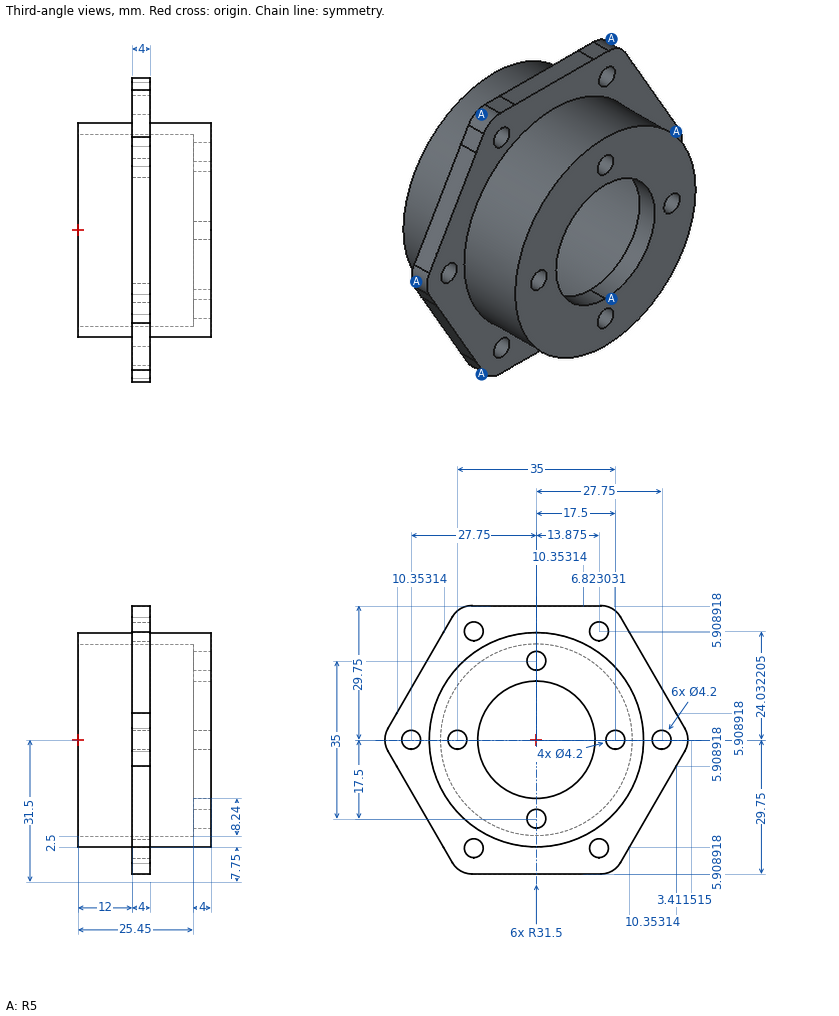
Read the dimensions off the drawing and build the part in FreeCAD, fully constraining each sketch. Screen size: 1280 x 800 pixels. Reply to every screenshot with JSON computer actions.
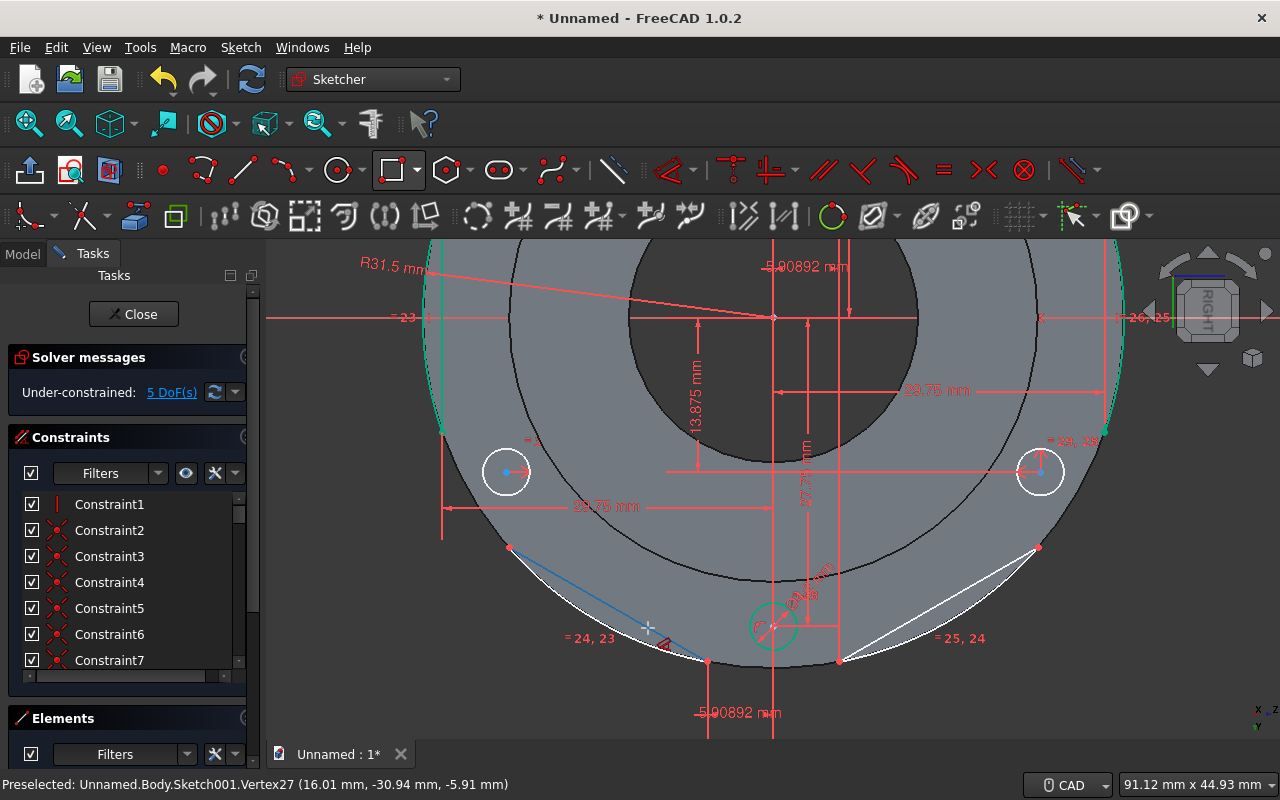
{"action": "left_click", "coordinate": [648, 628]}
{"action": "left_click", "coordinate": [475, 605]}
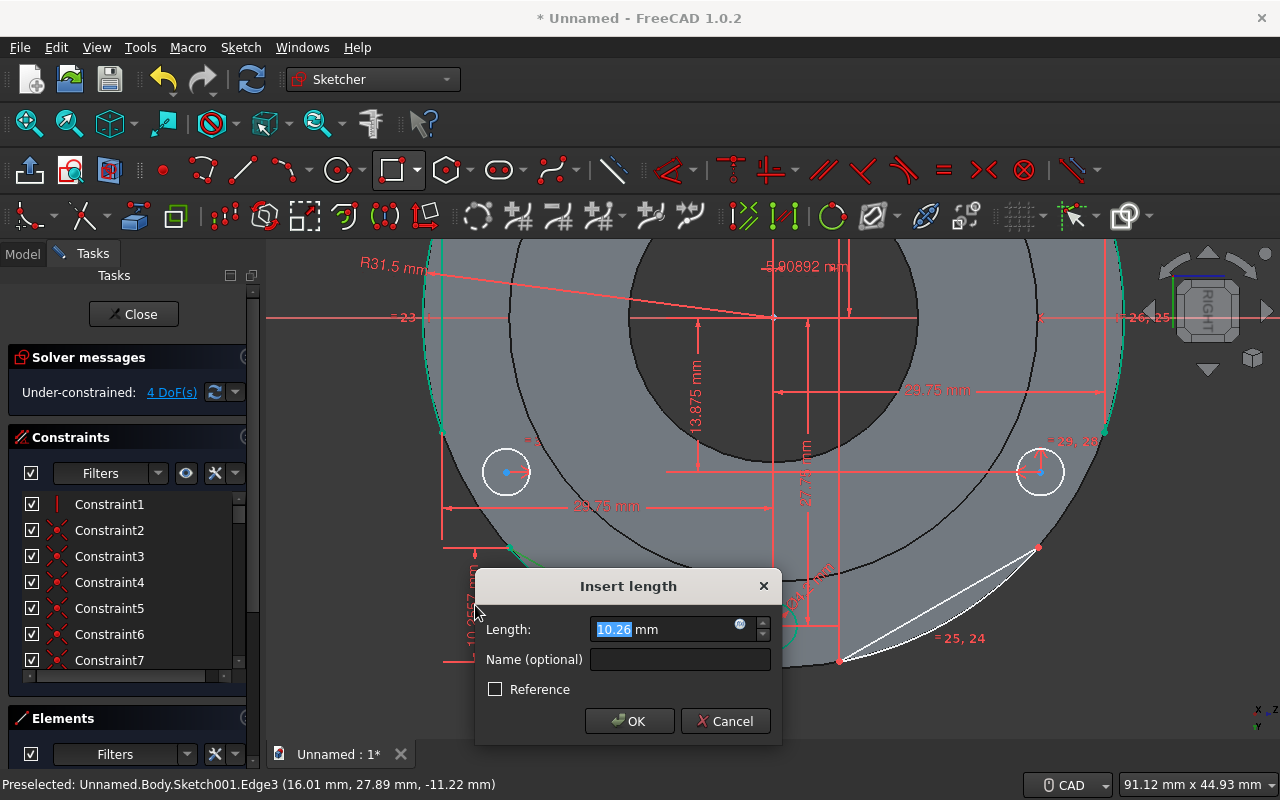
{"action": "type", "text": "10.35314"}
{"action": "key", "text": "Return"}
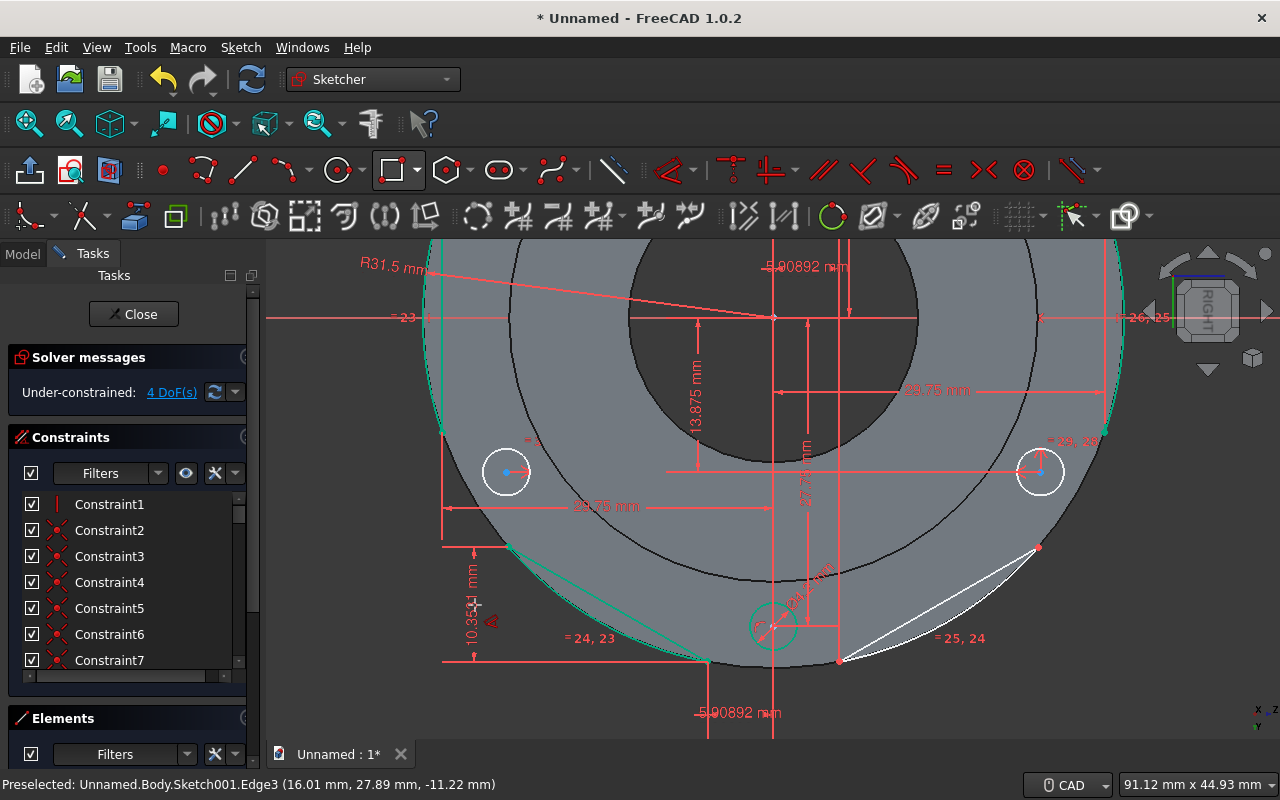
{"action": "left_click", "coordinate": [978, 582]}
{"action": "left_click", "coordinate": [1072, 605]}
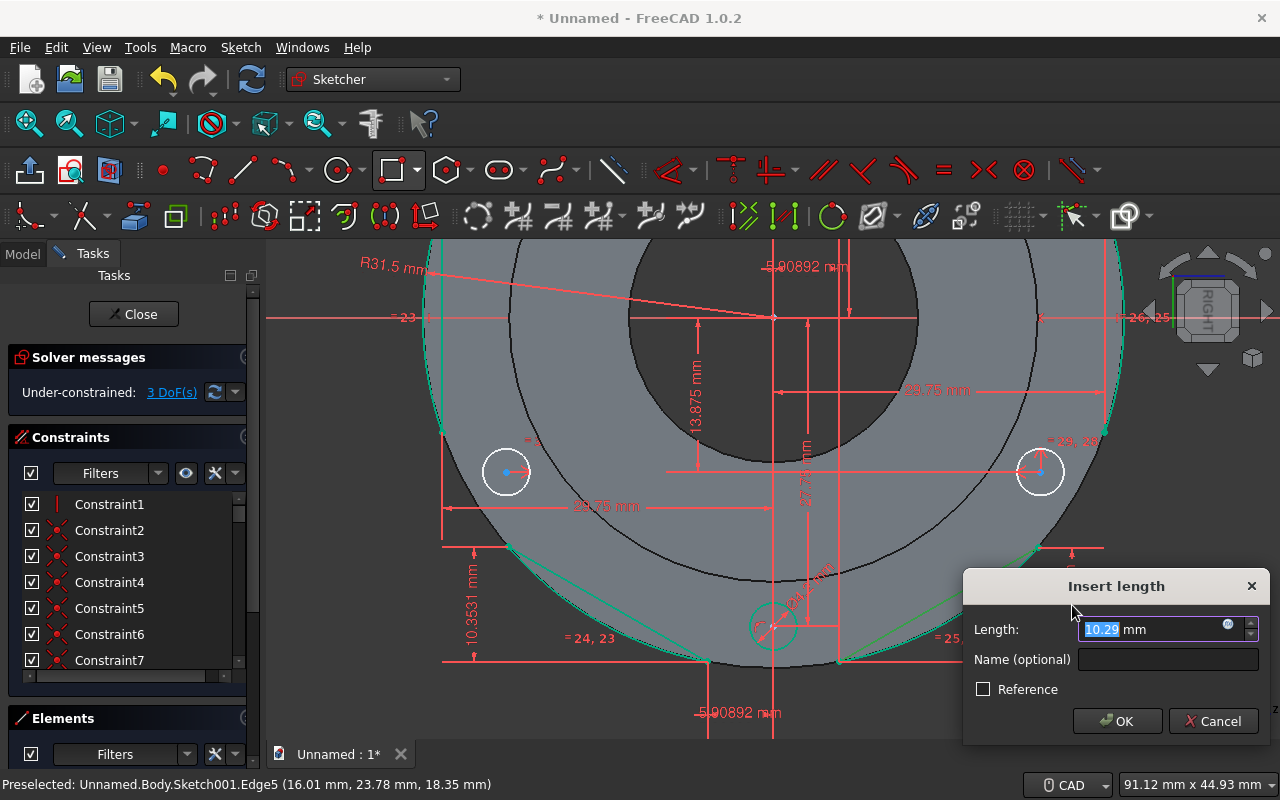
{"action": "type", "text": "10.35314"}
{"action": "key", "text": "Return"}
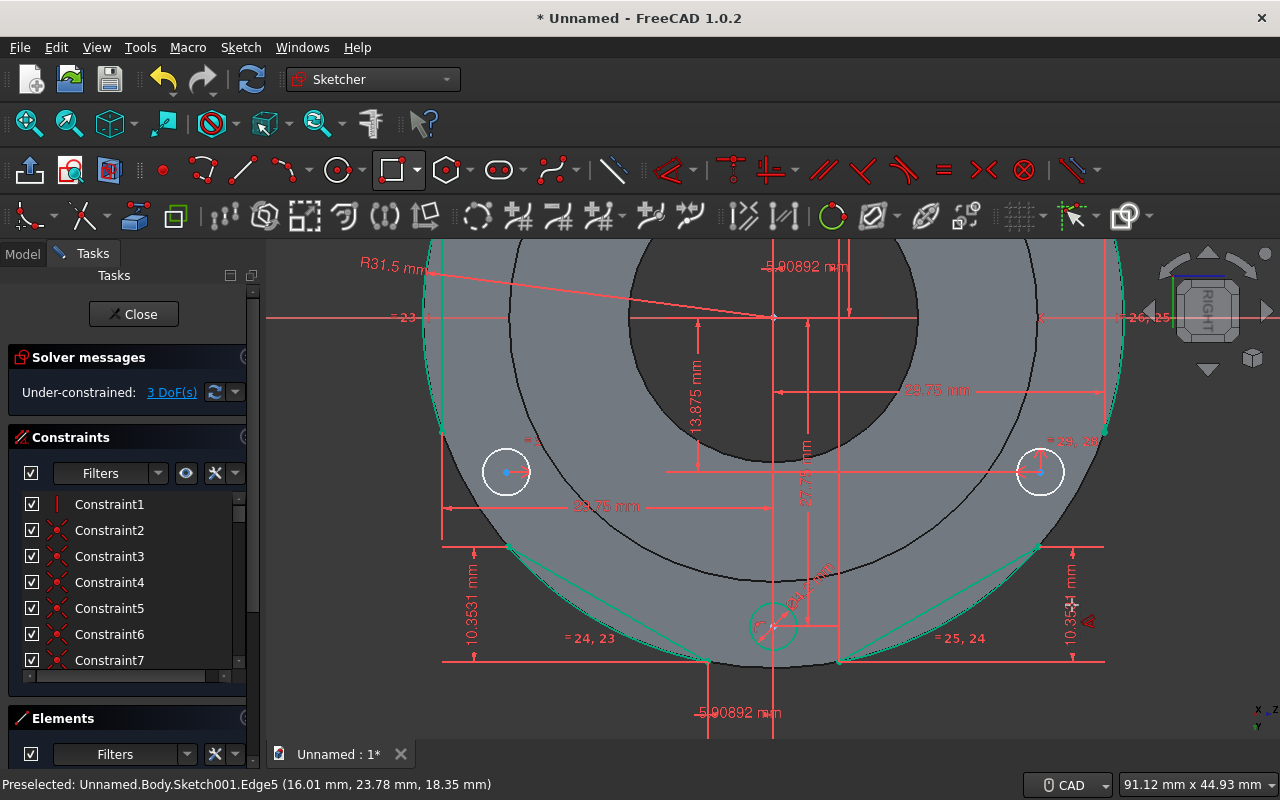
{"action": "scroll", "coordinate": [648, 629], "scroll_direction": "down", "scroll_amount": 4}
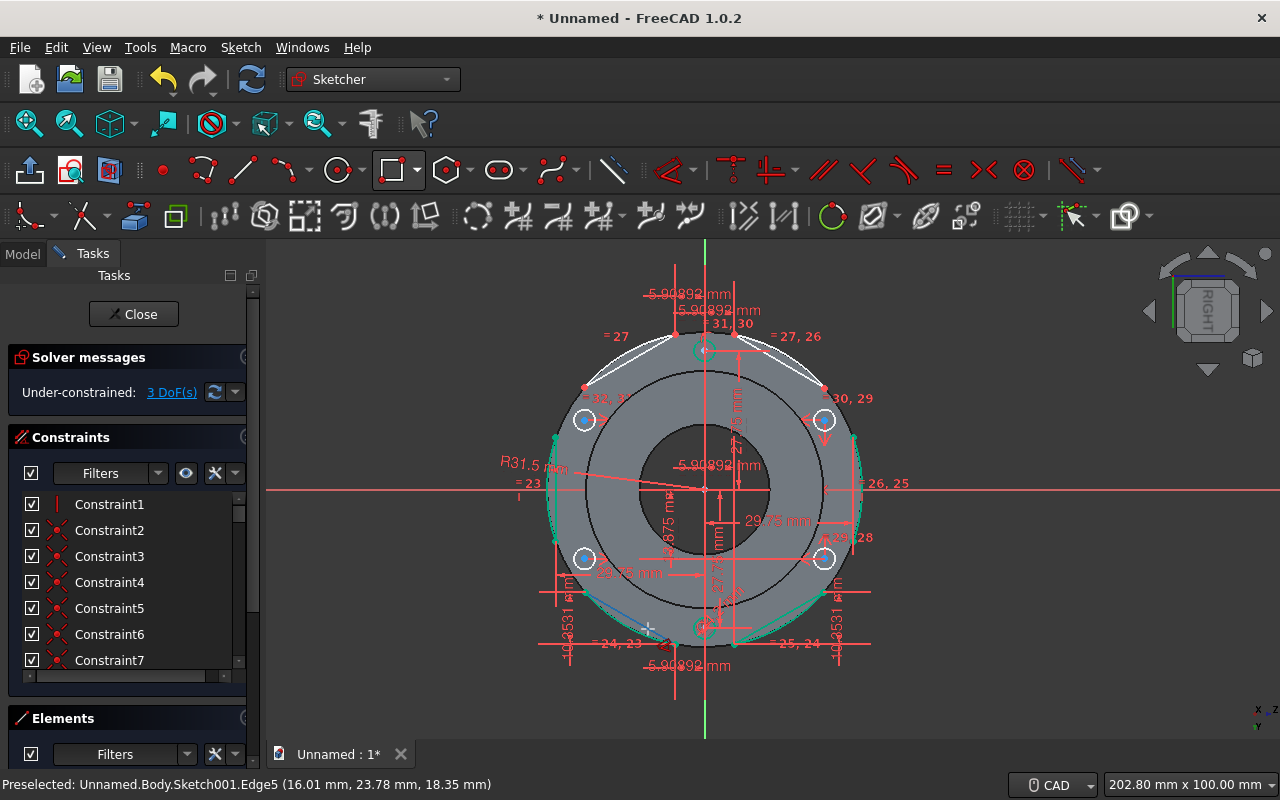
{"action": "scroll", "coordinate": [761, 351], "scroll_direction": "up", "scroll_amount": 4}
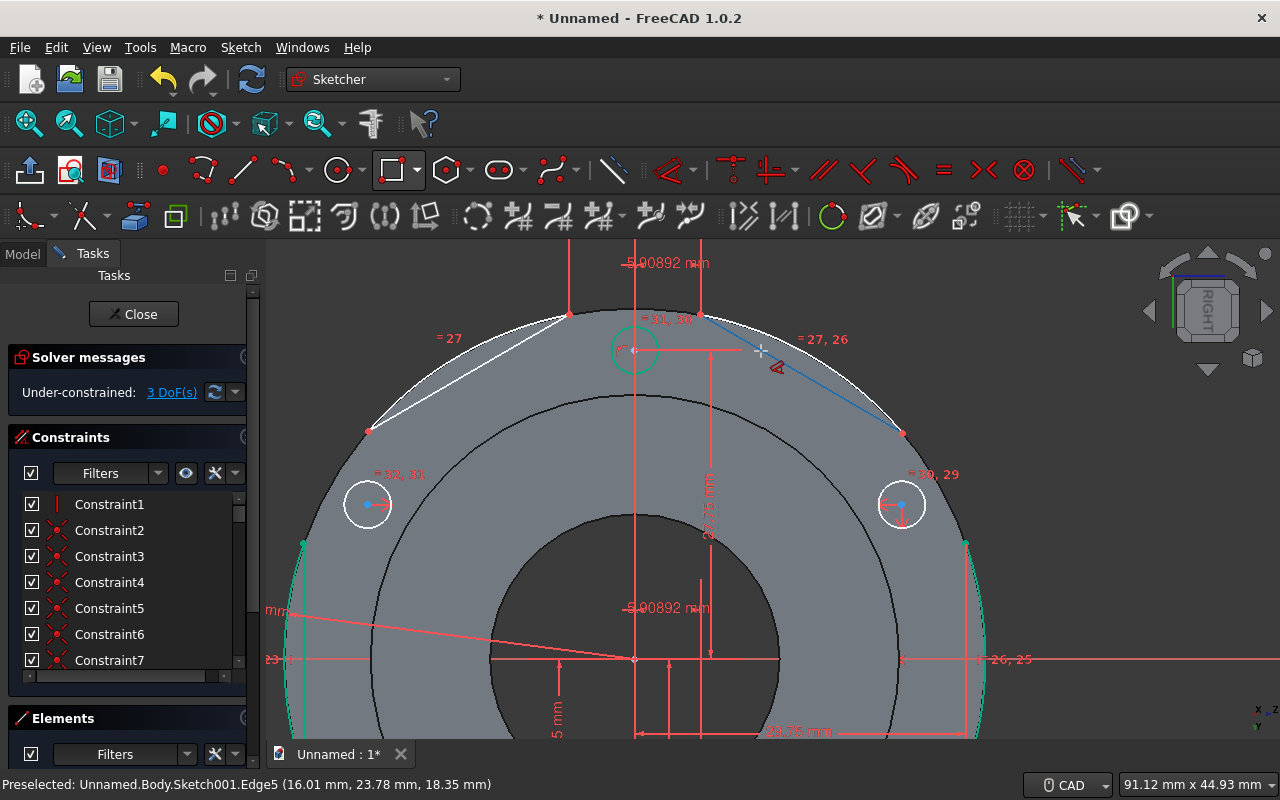
{"action": "left_click", "coordinate": [761, 350]}
{"action": "left_click", "coordinate": [937, 374]}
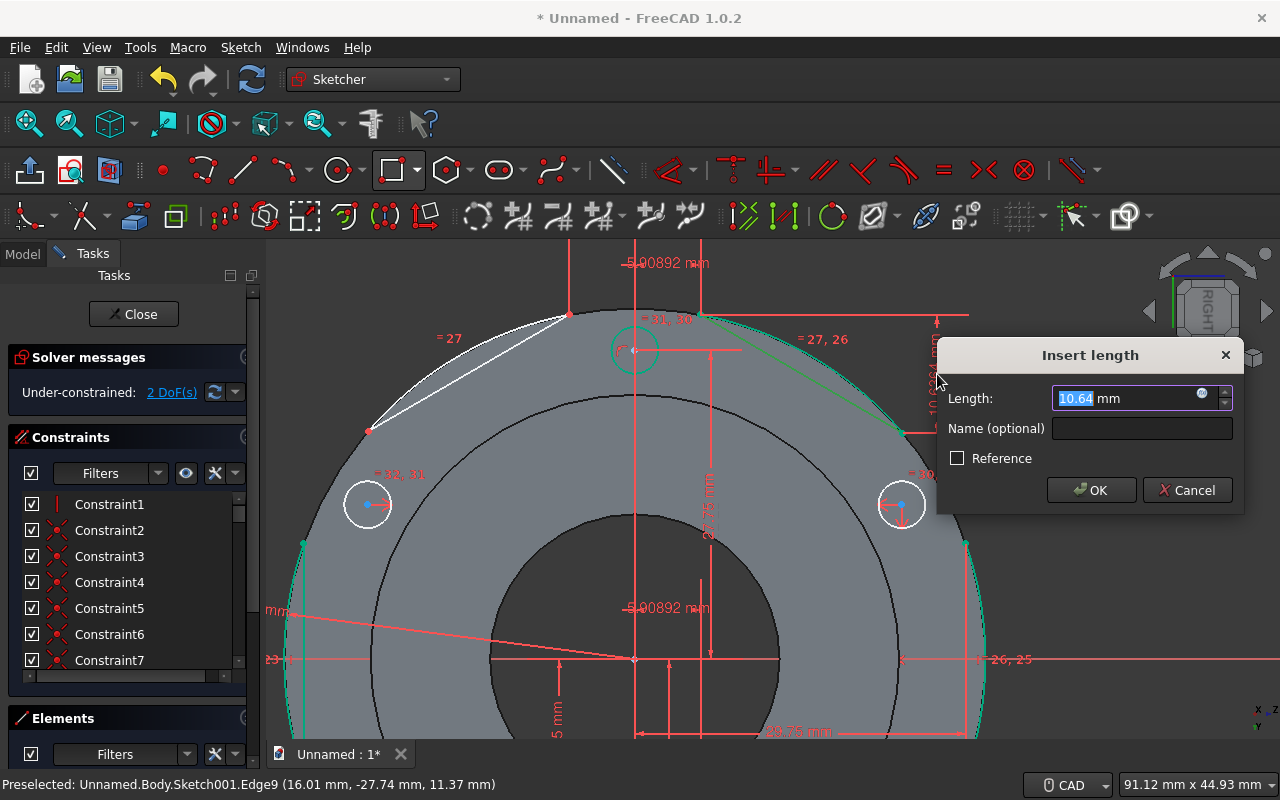
{"action": "type", "text": "10.35314"}
{"action": "key", "text": "Return"}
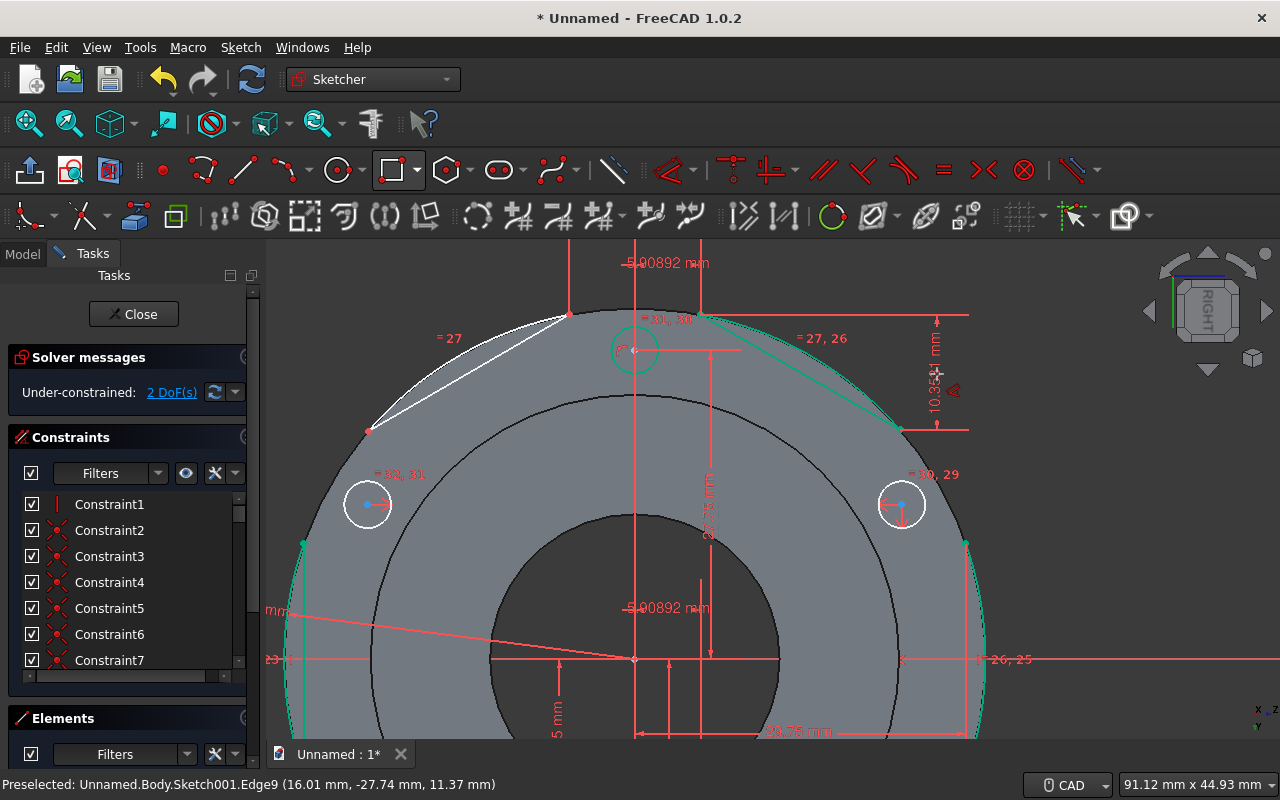
{"action": "left_click", "coordinate": [429, 396]}
{"action": "left_click", "coordinate": [335, 373]}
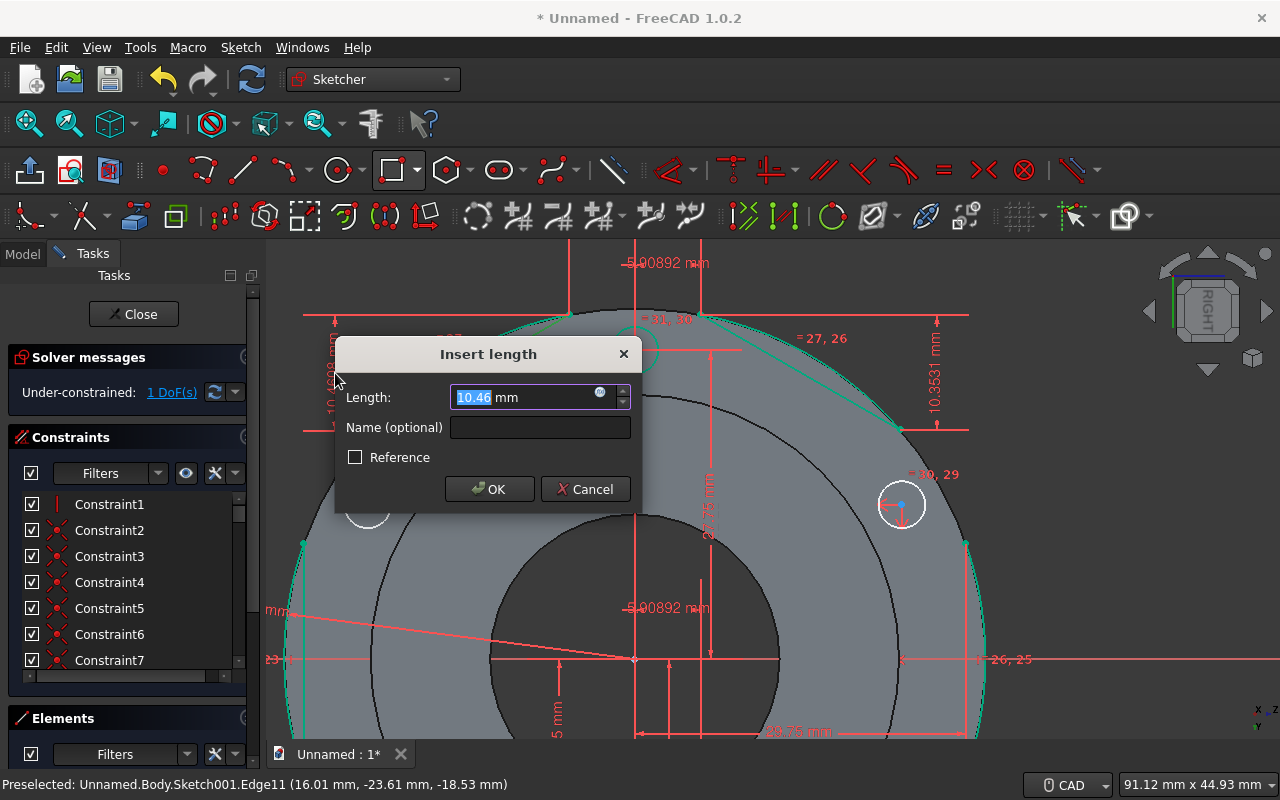
{"action": "type", "text": "10.35314"}
{"action": "key", "text": "Return"}